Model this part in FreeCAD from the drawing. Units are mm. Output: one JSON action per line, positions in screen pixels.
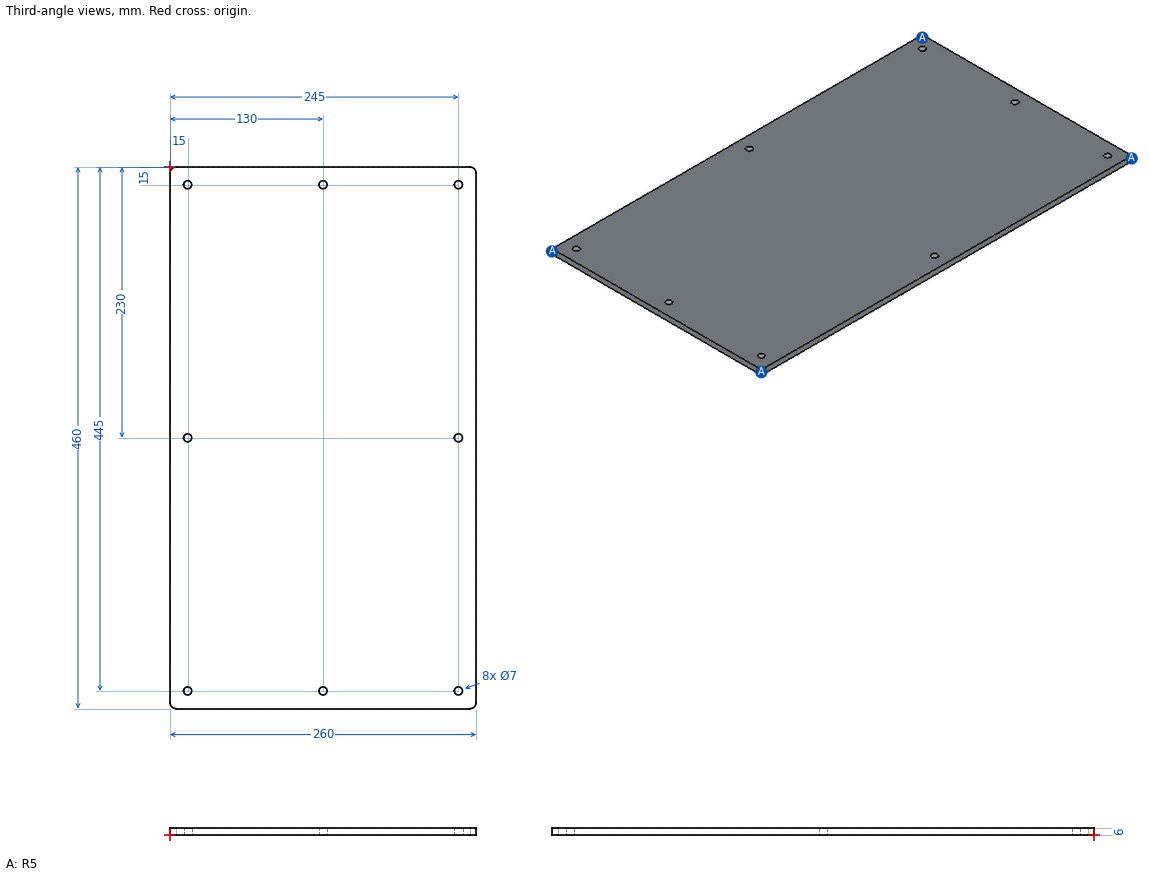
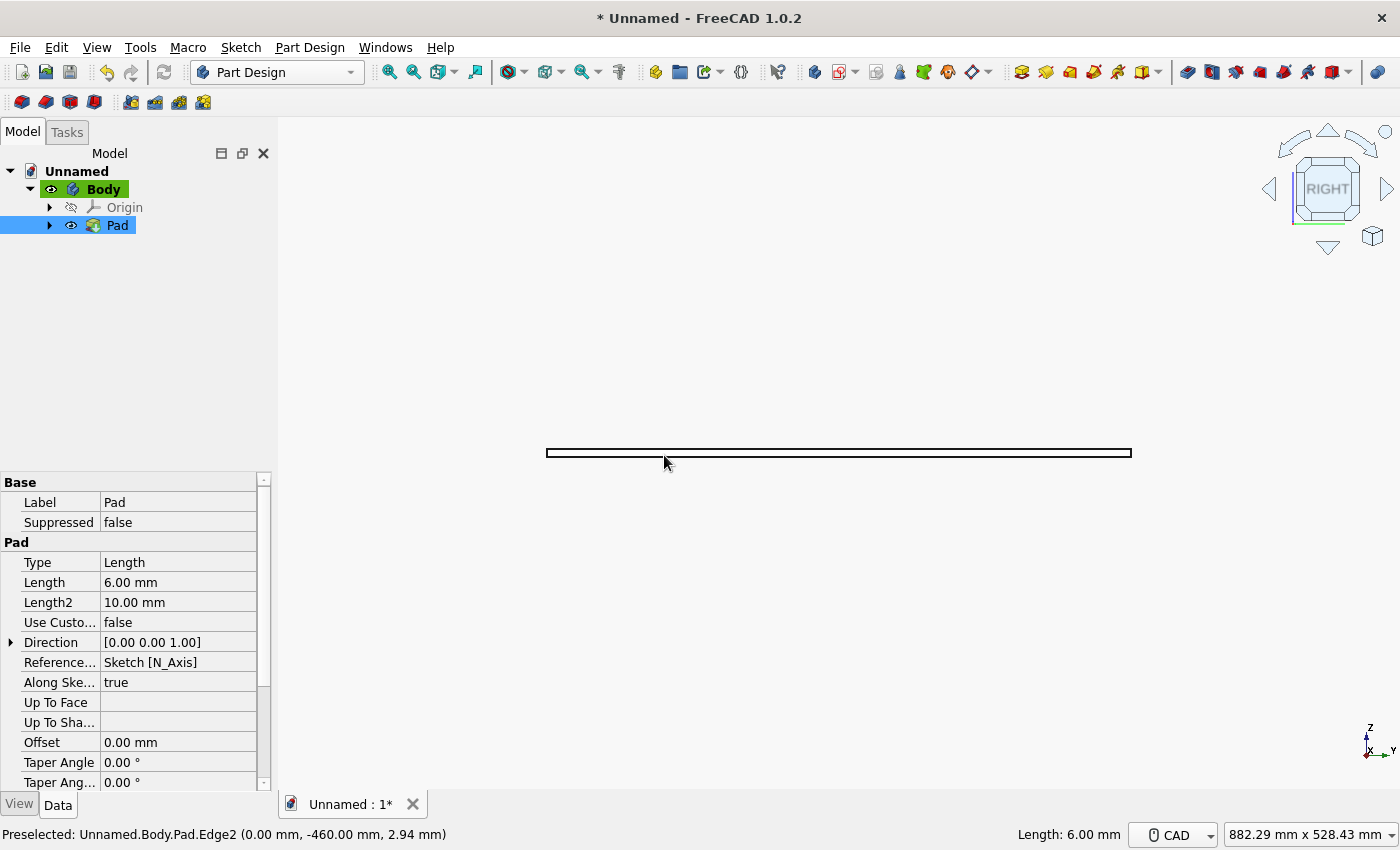
{"action": "scroll", "coordinate": [1131, 452], "scroll_direction": "up", "scroll_amount": 9}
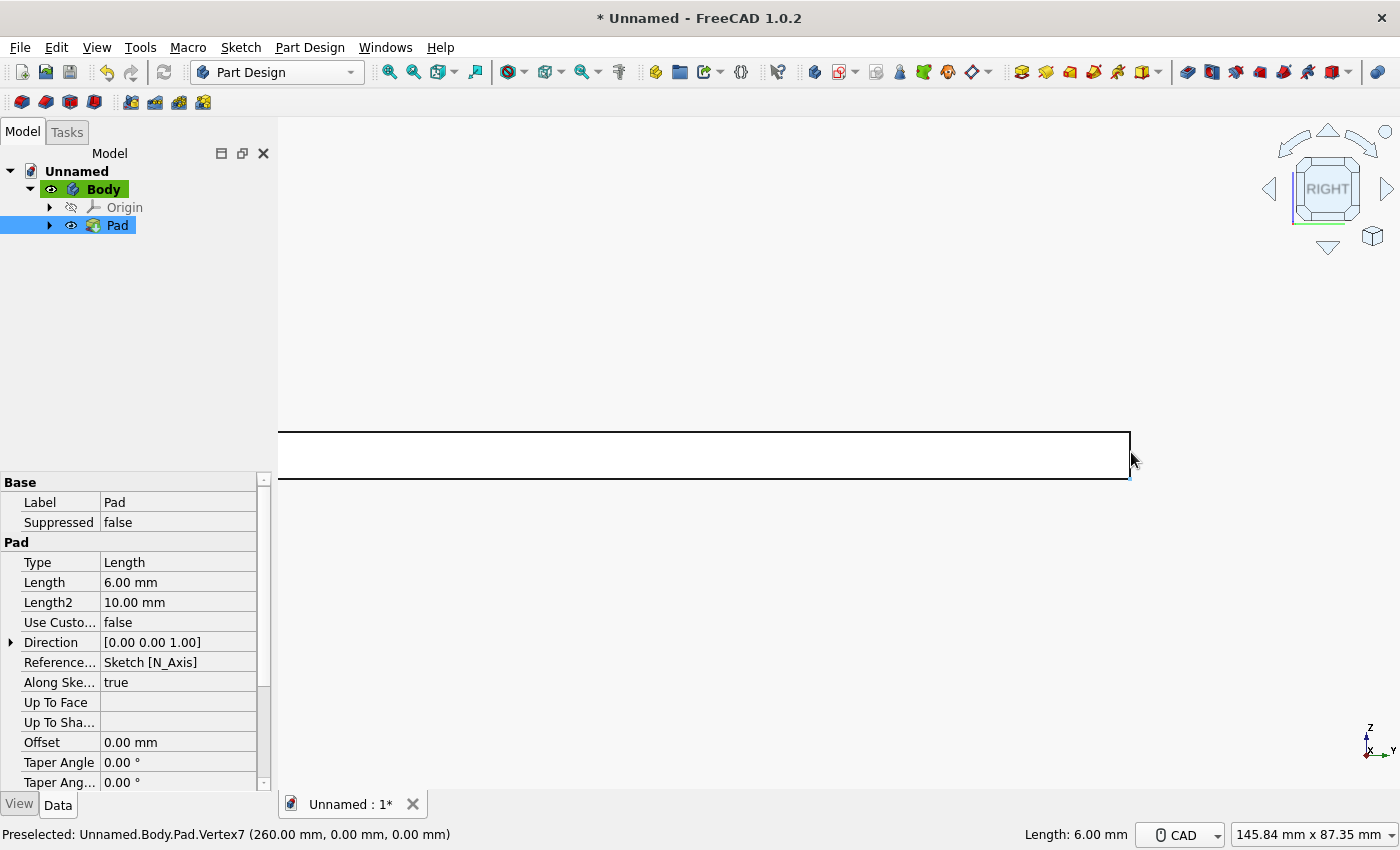
{"action": "left_click", "coordinate": [1130, 455], "text": "ctrl"}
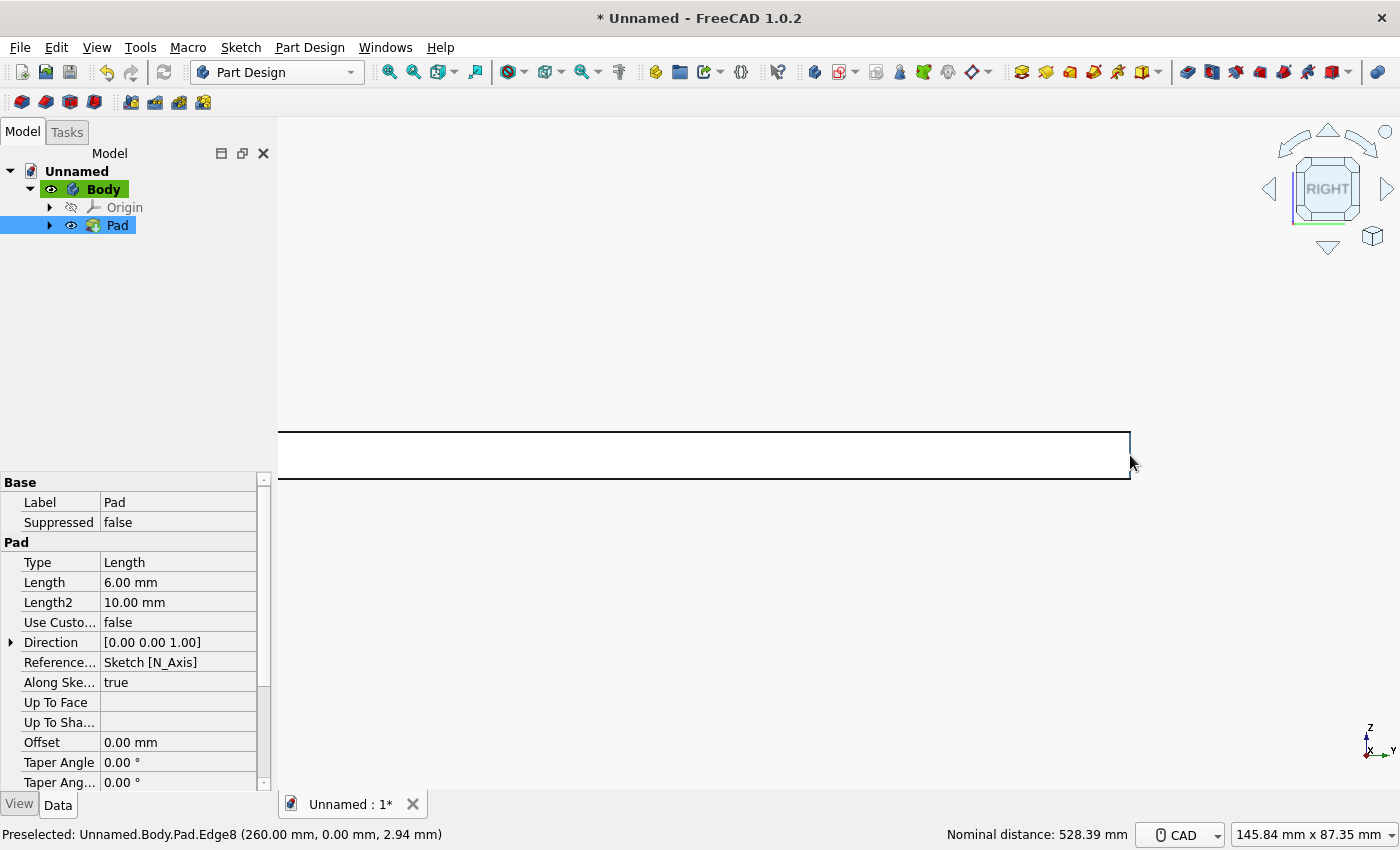
{"action": "left_click", "coordinate": [390, 72]}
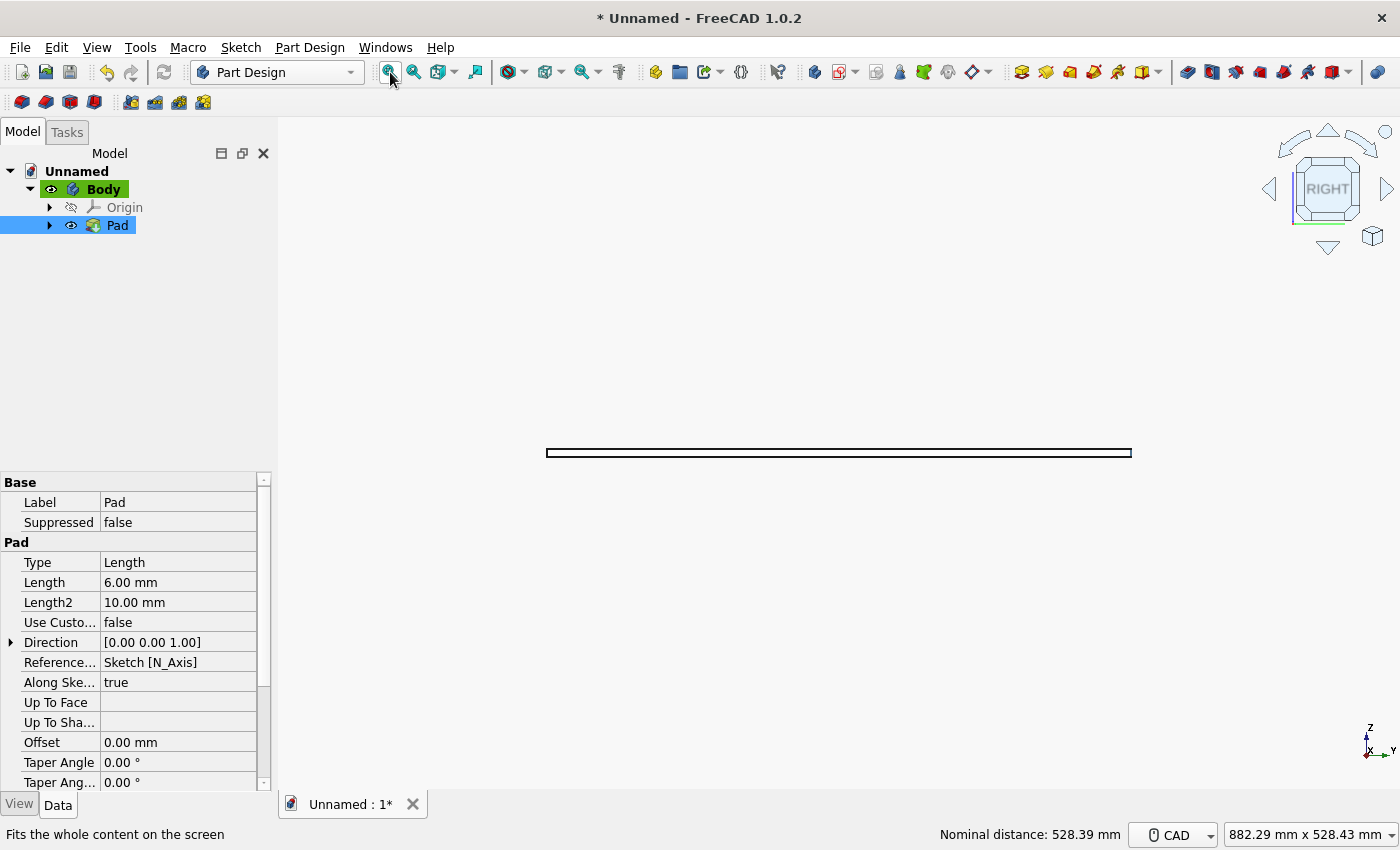
{"action": "key", "text": "5"}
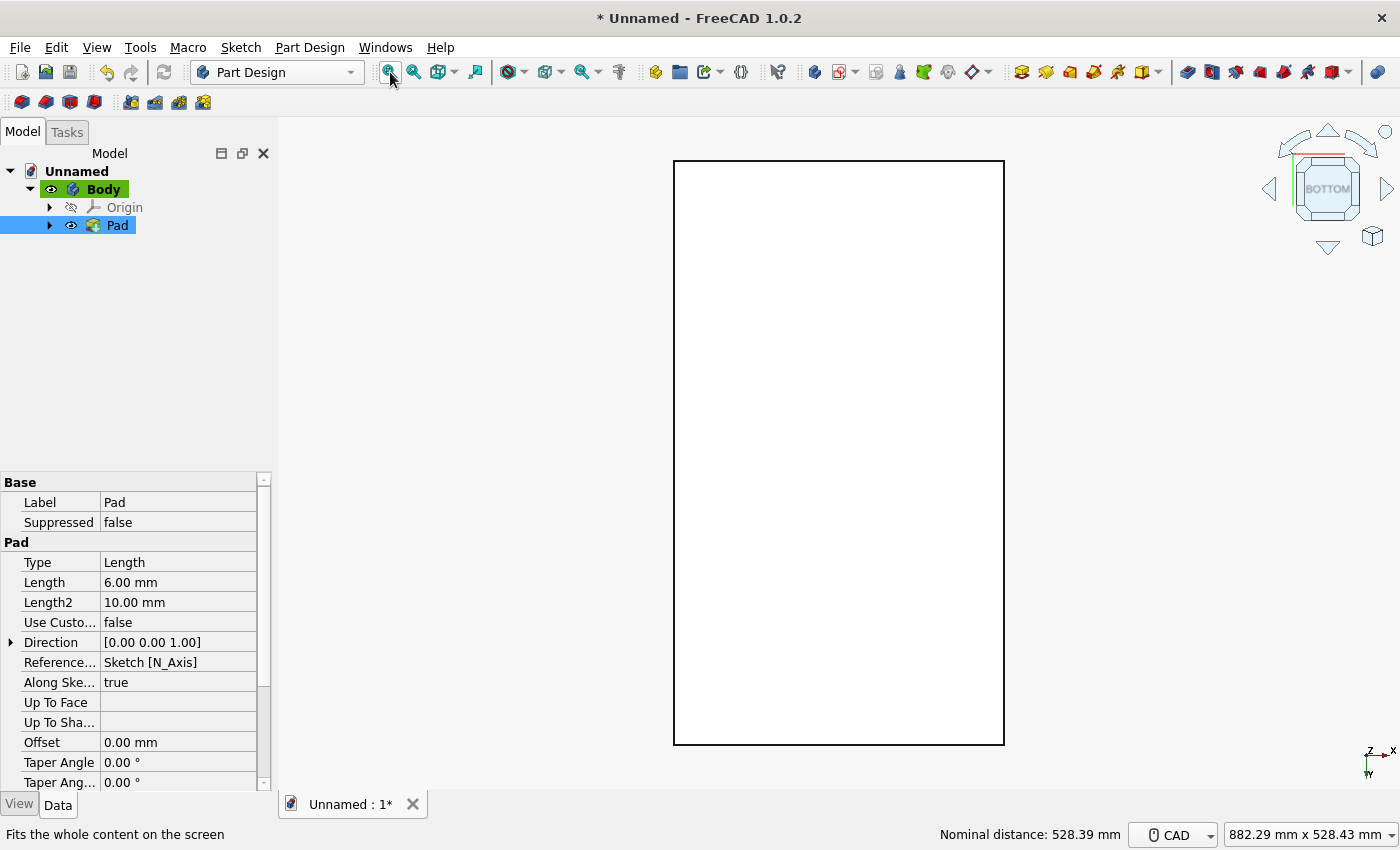
{"action": "scroll", "coordinate": [674, 744], "scroll_direction": "up", "scroll_amount": 9}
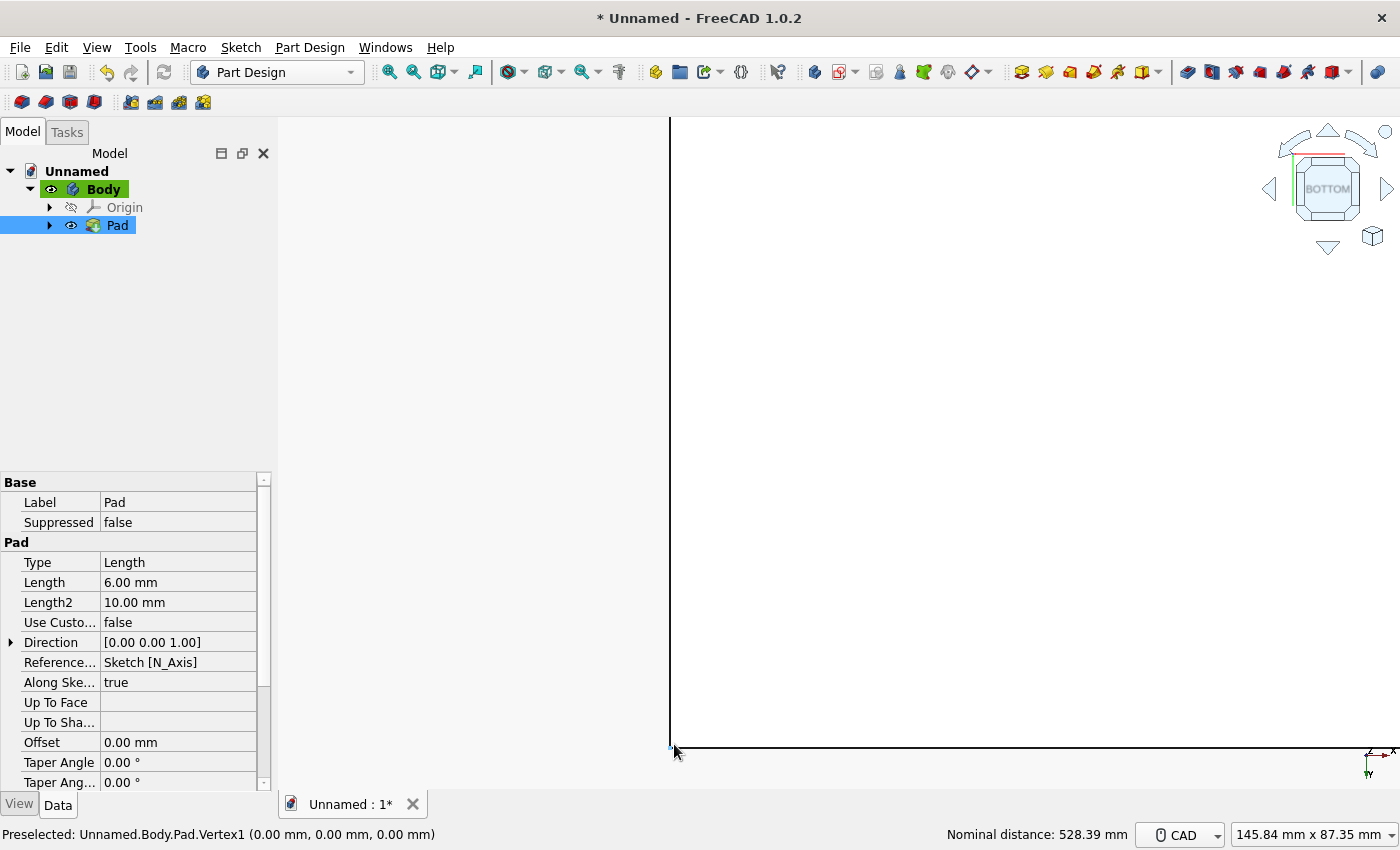
{"action": "left_click", "coordinate": [390, 72]}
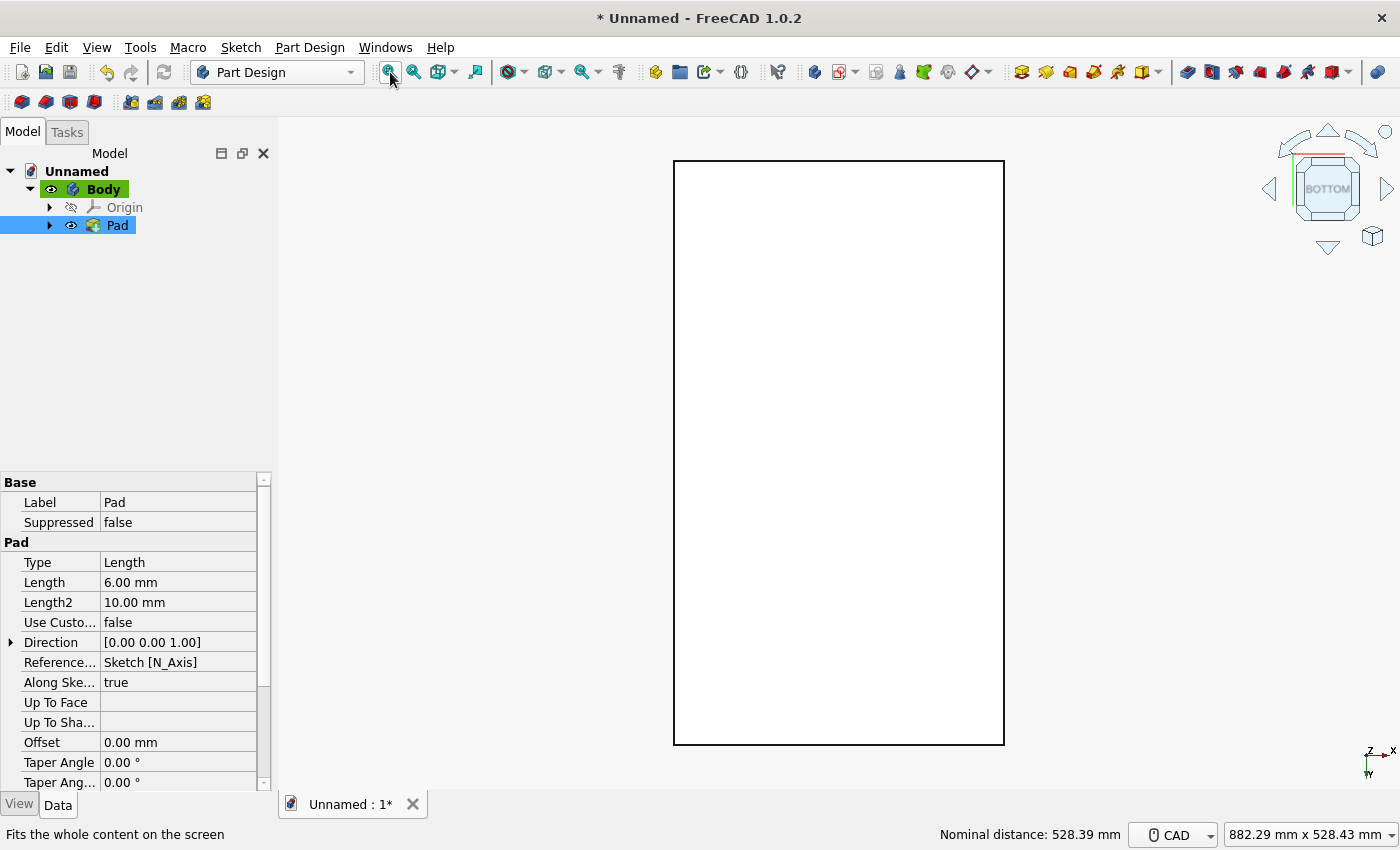
{"action": "key", "text": "4"}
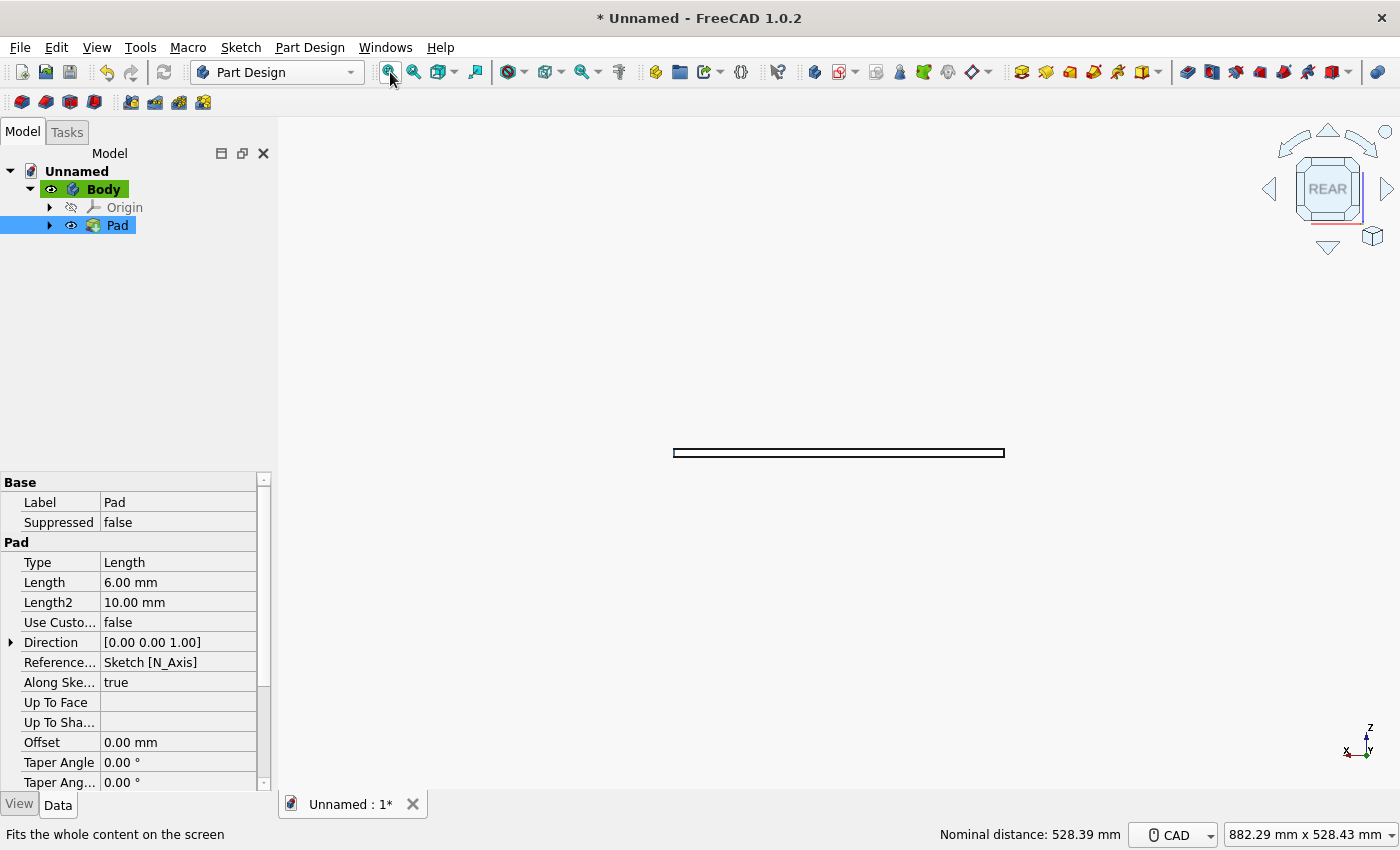
{"action": "left_click", "coordinate": [390, 72]}